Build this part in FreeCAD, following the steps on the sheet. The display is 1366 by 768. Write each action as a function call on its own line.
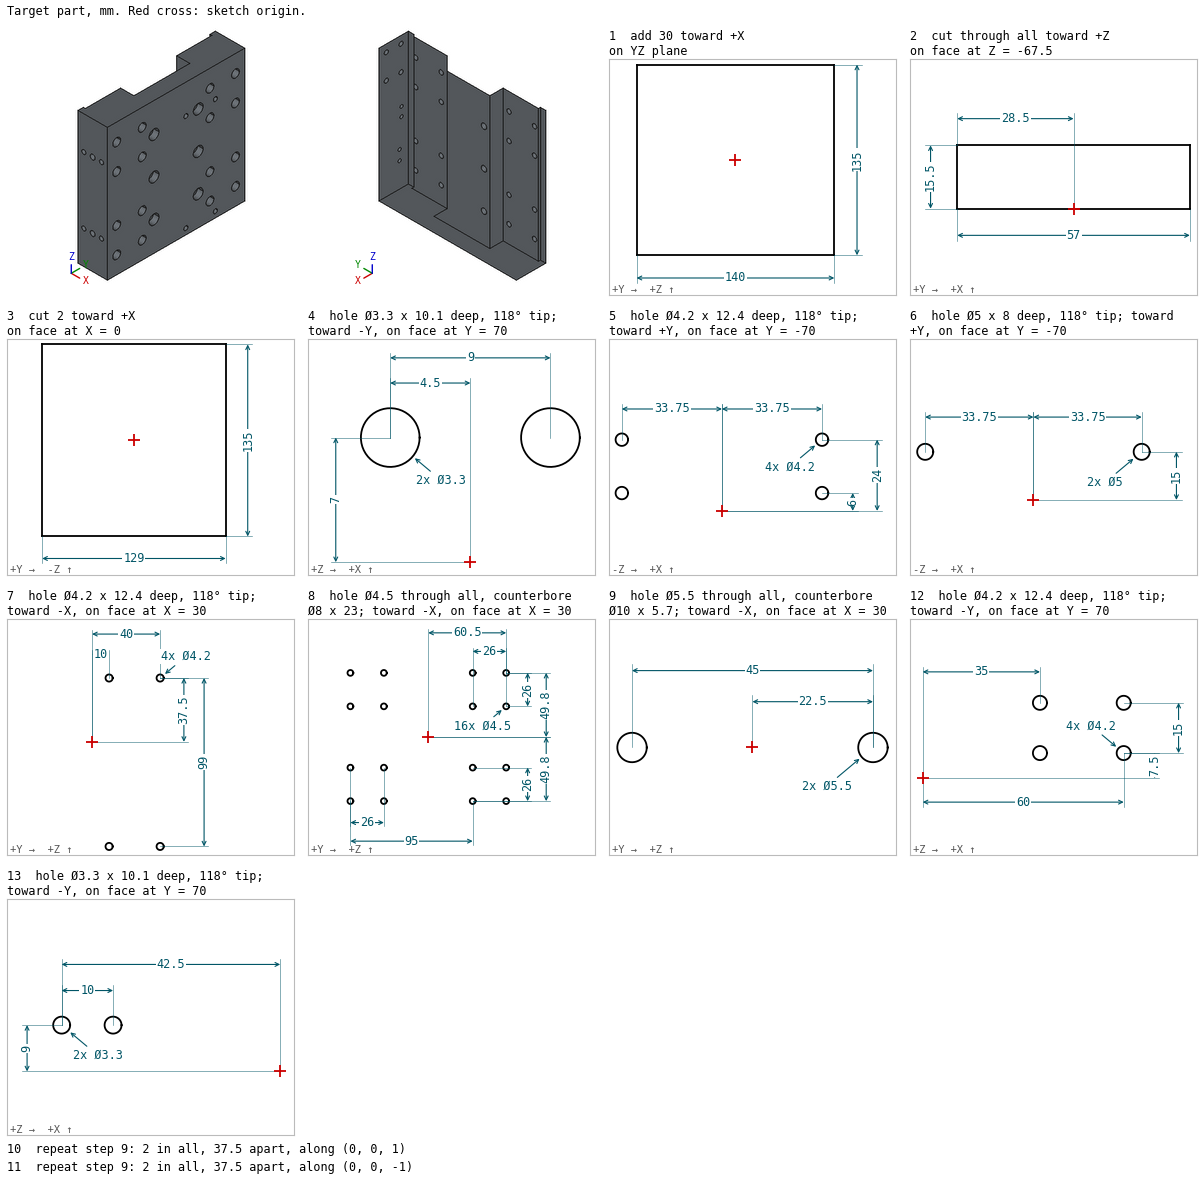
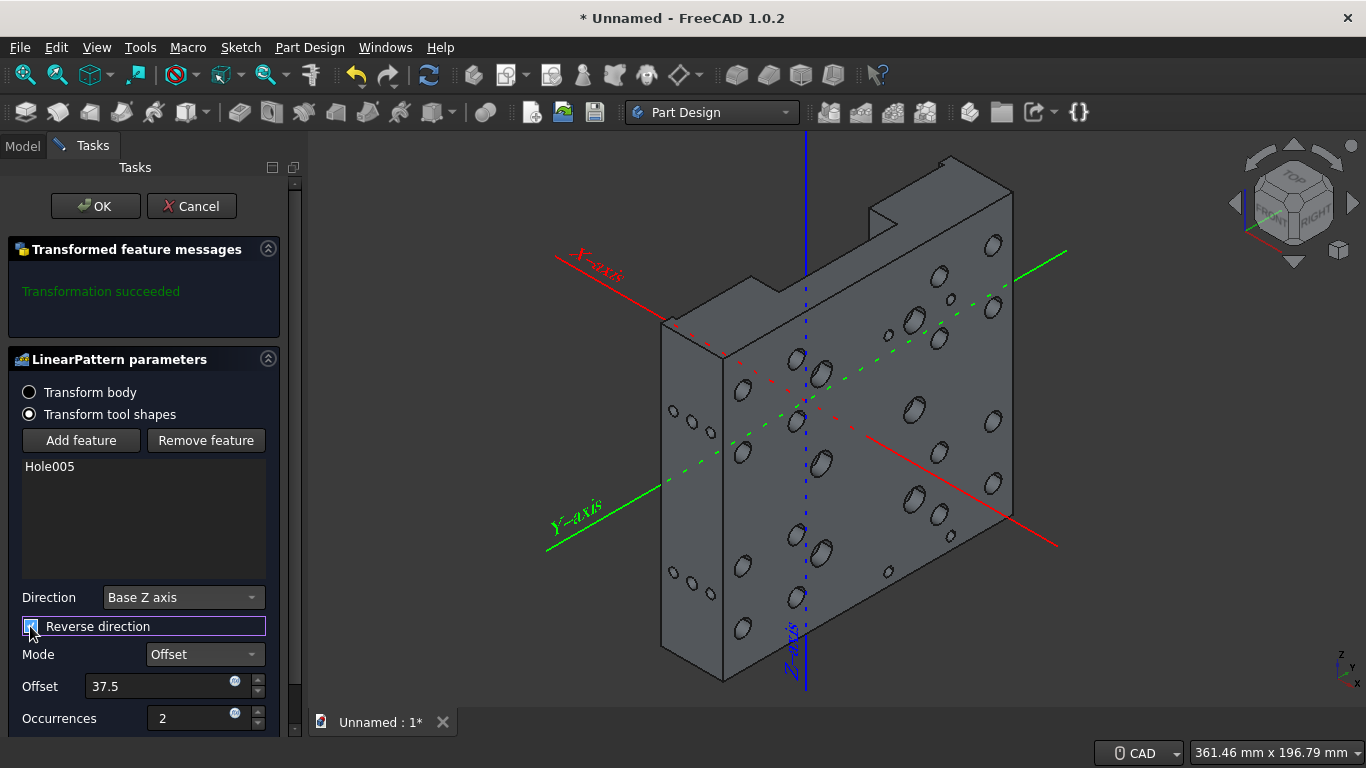
click(96, 206)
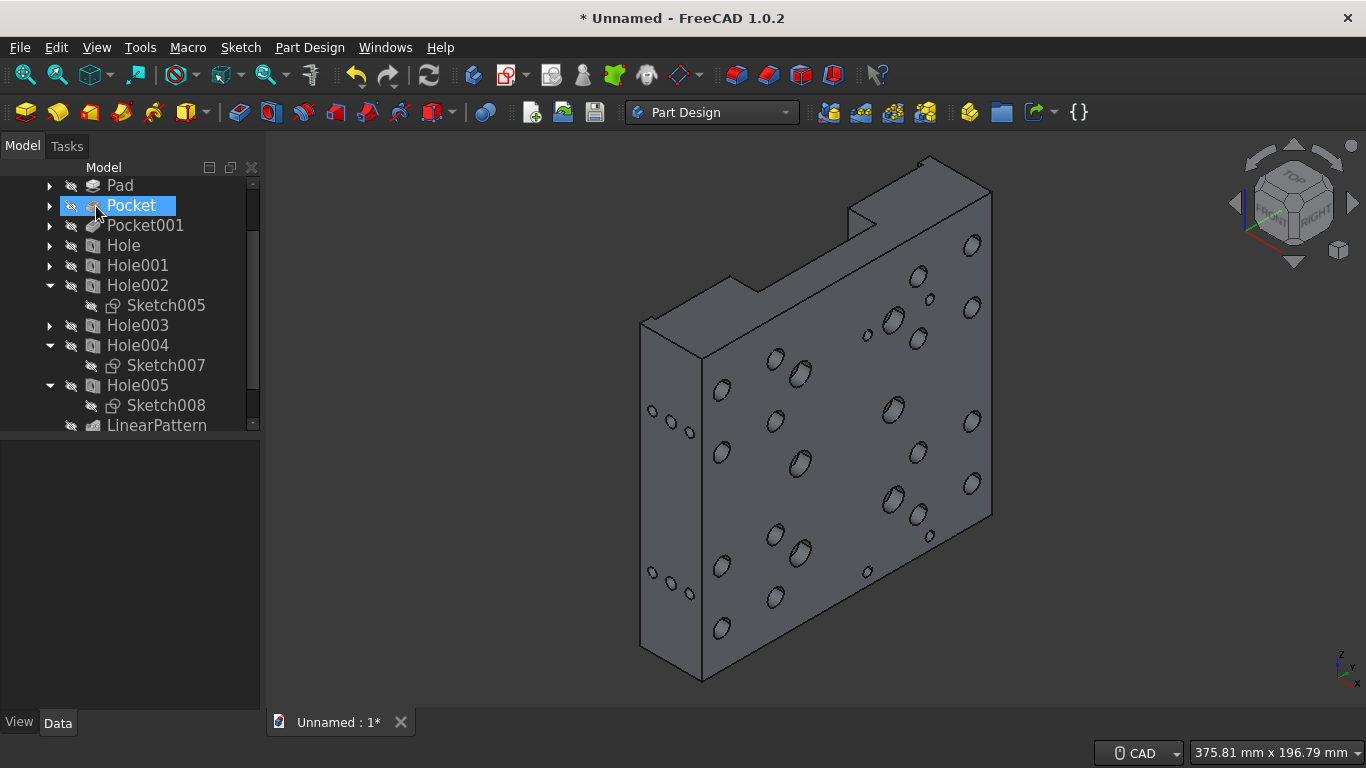
key(4)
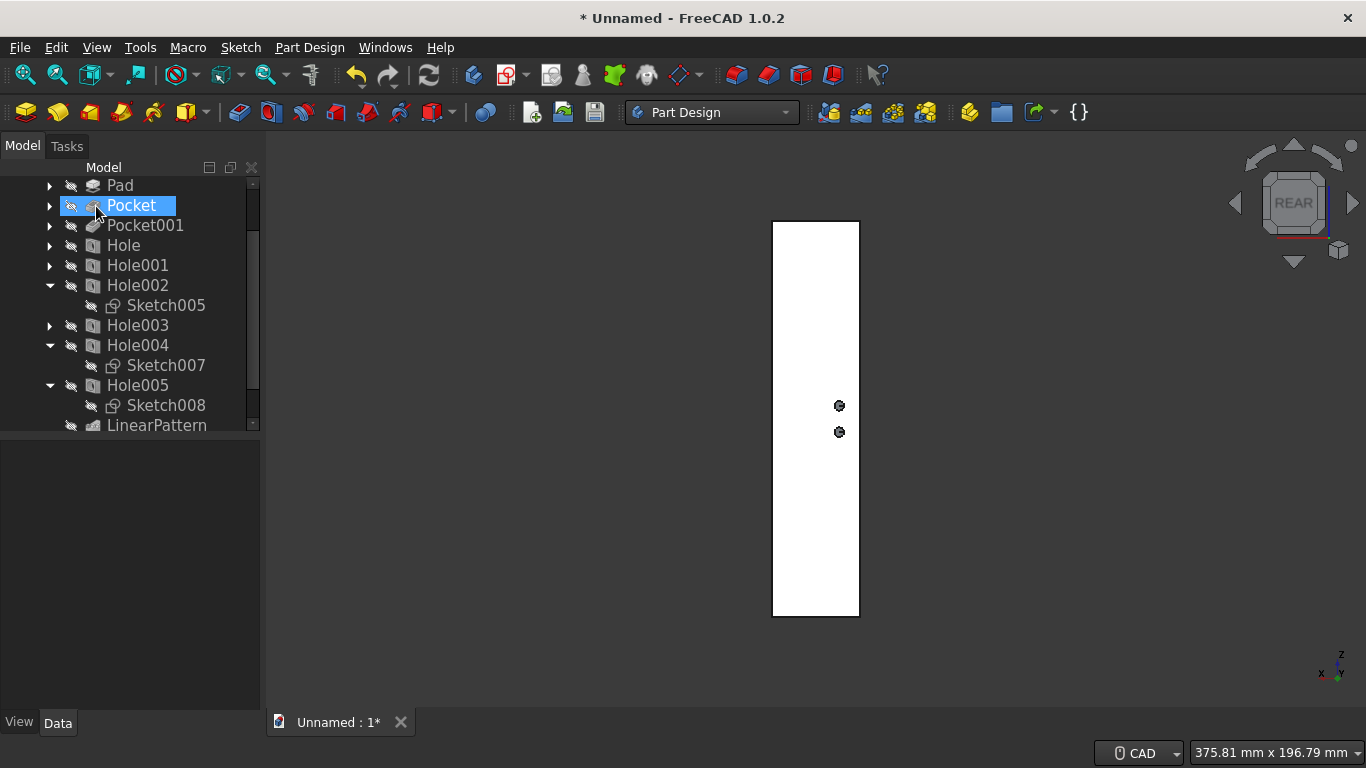
click(816, 362)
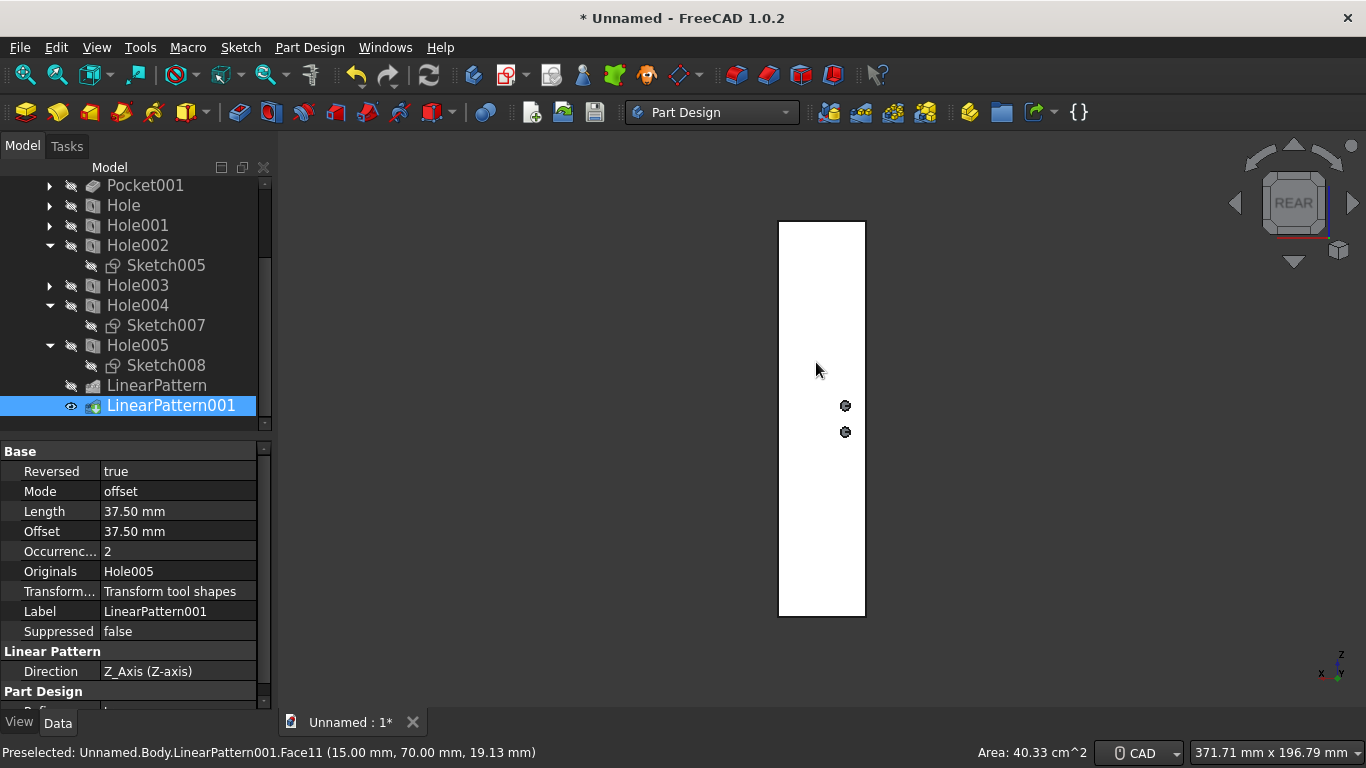
click(506, 76)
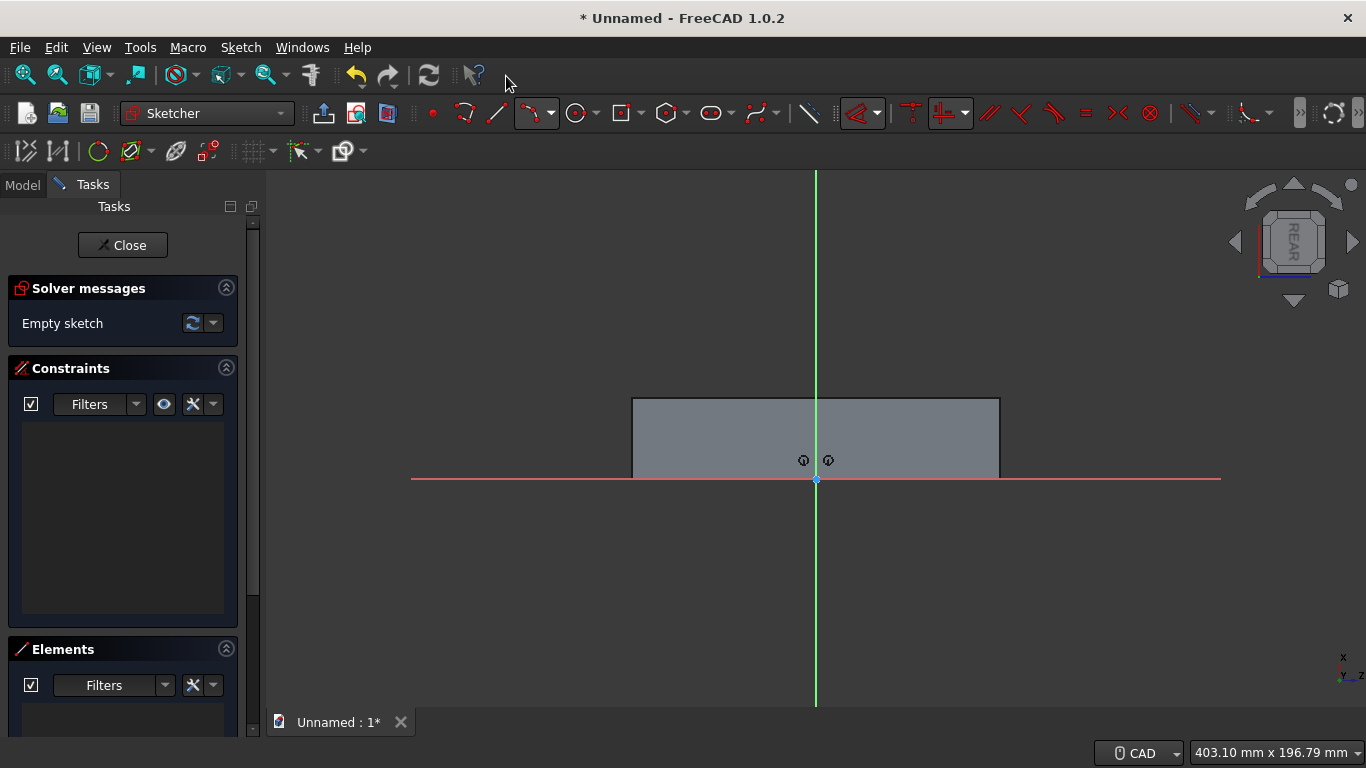
scroll(951, 448, up, 7)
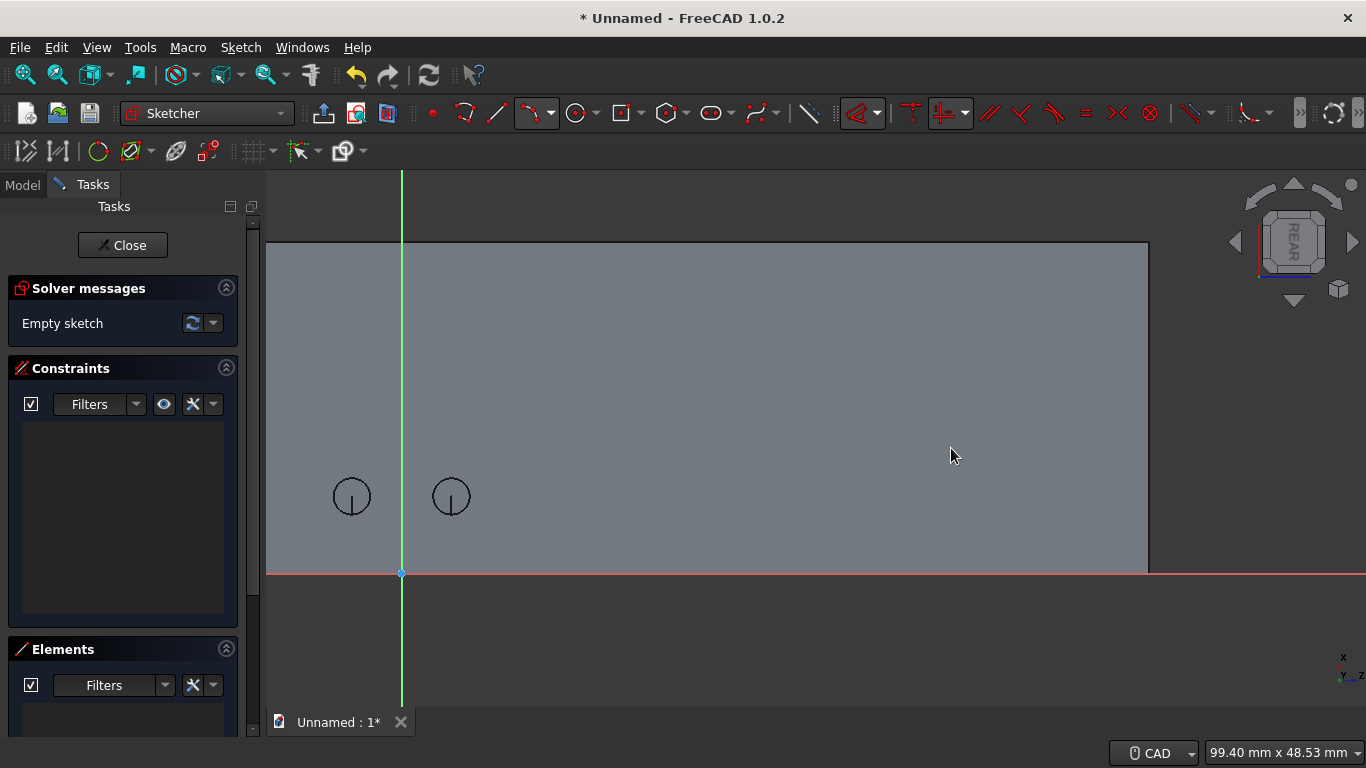
click(576, 114)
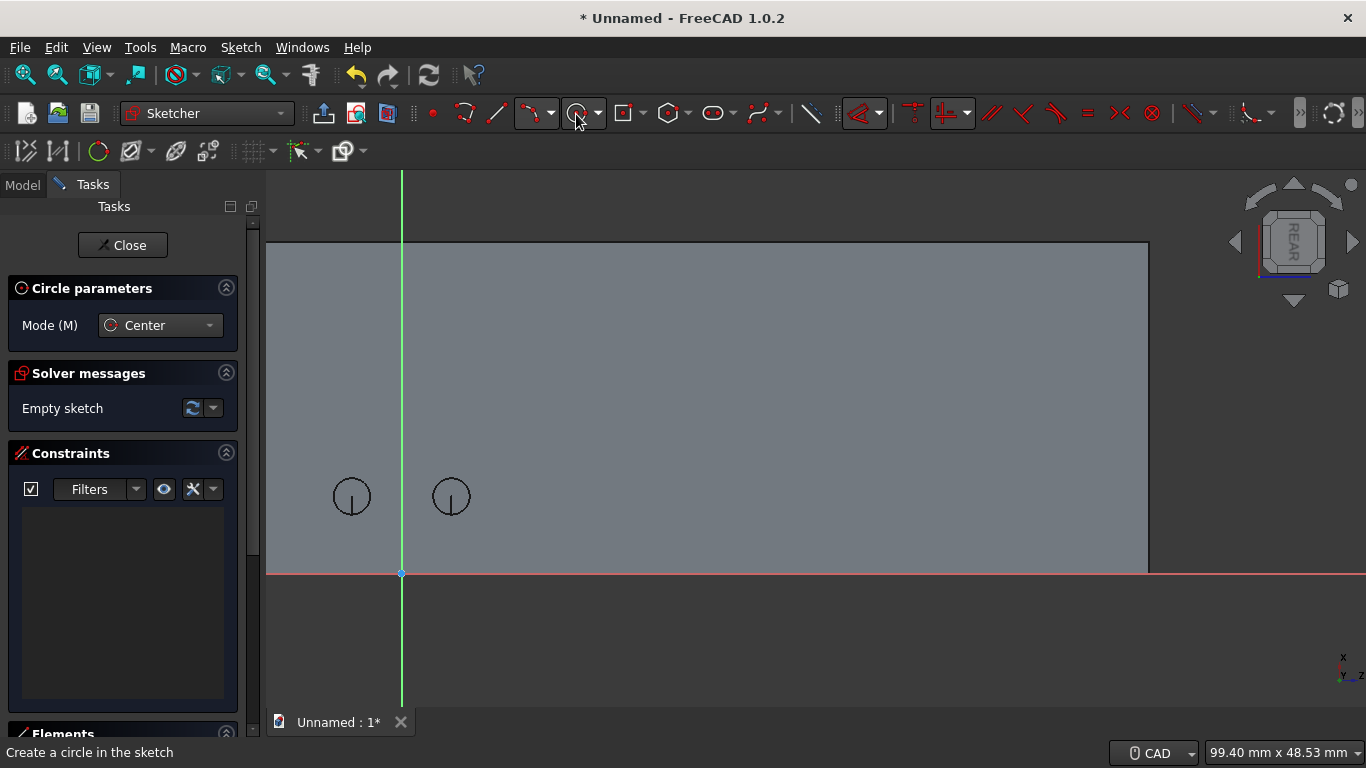
click(1066, 491)
click(1082, 474)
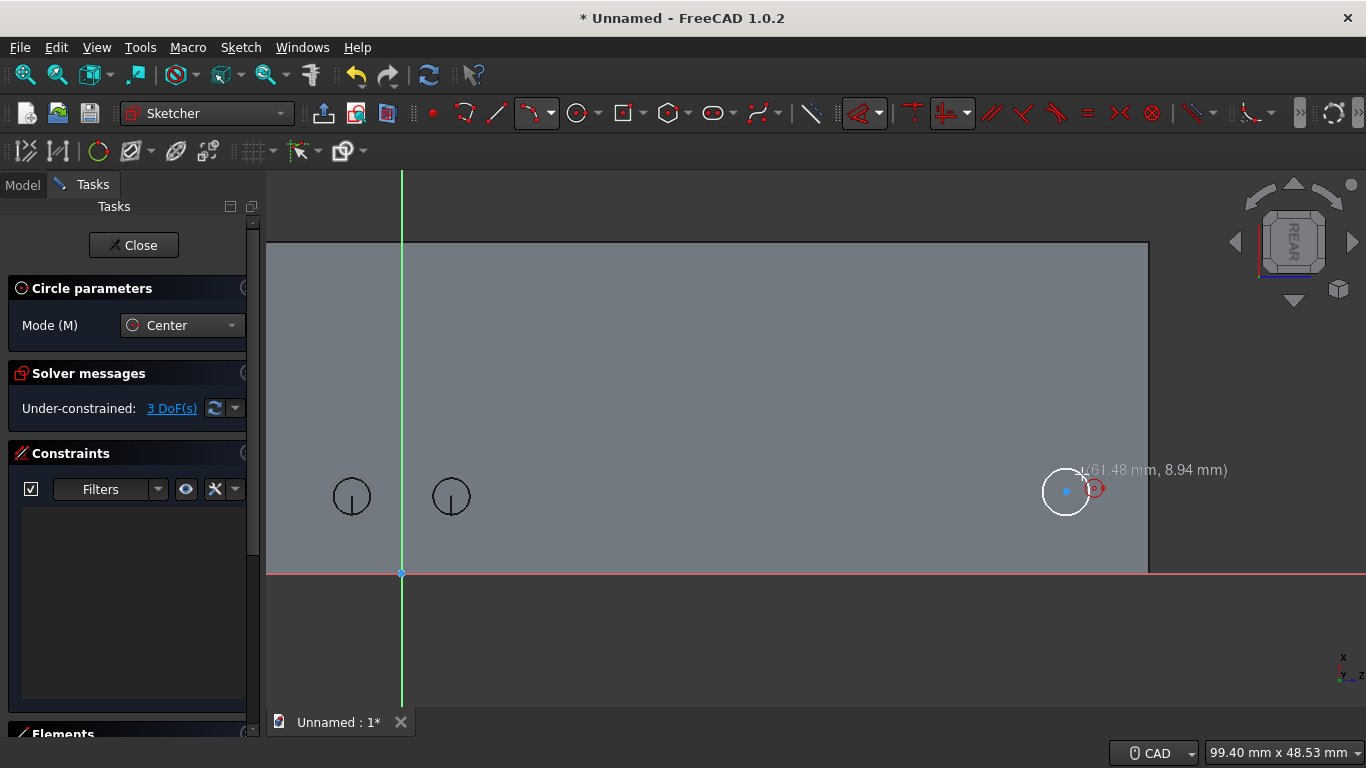
click(1066, 325)
click(1082, 308)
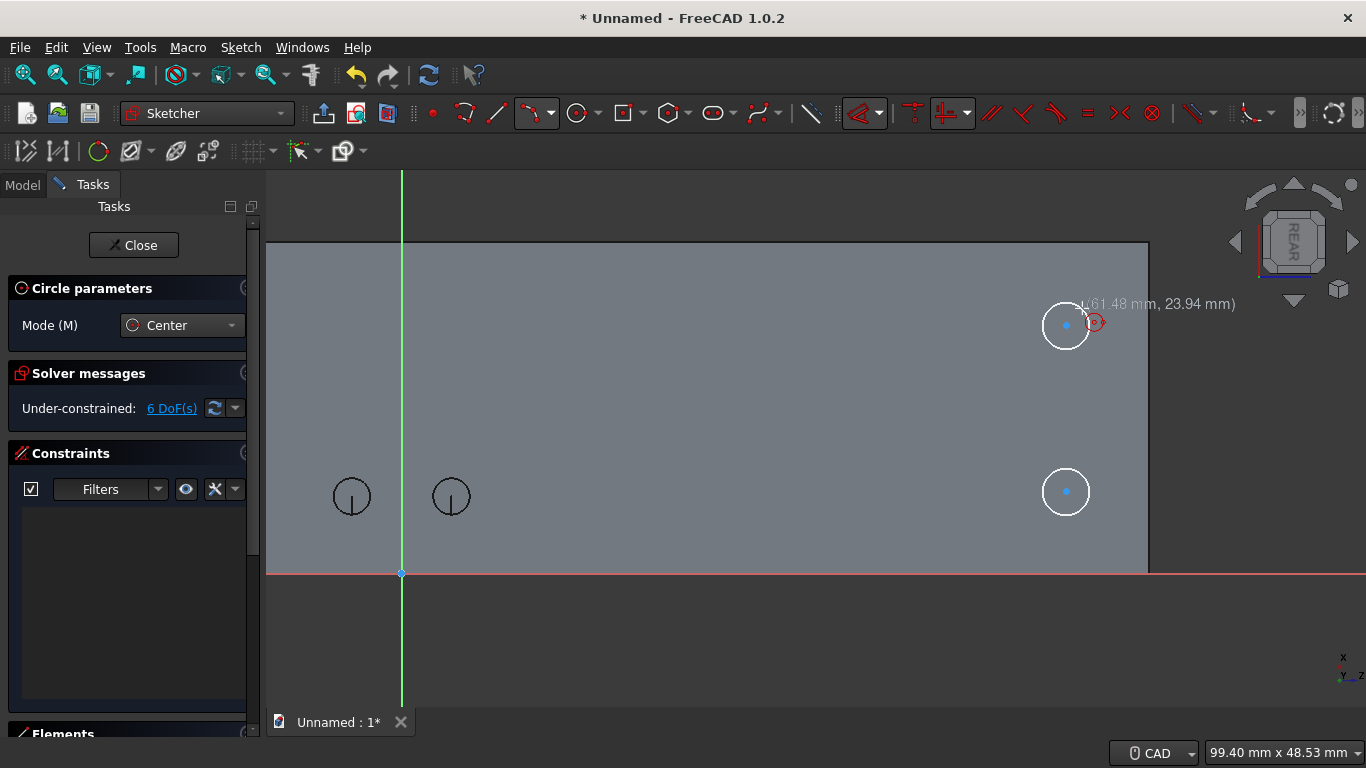
click(789, 325)
click(805, 308)